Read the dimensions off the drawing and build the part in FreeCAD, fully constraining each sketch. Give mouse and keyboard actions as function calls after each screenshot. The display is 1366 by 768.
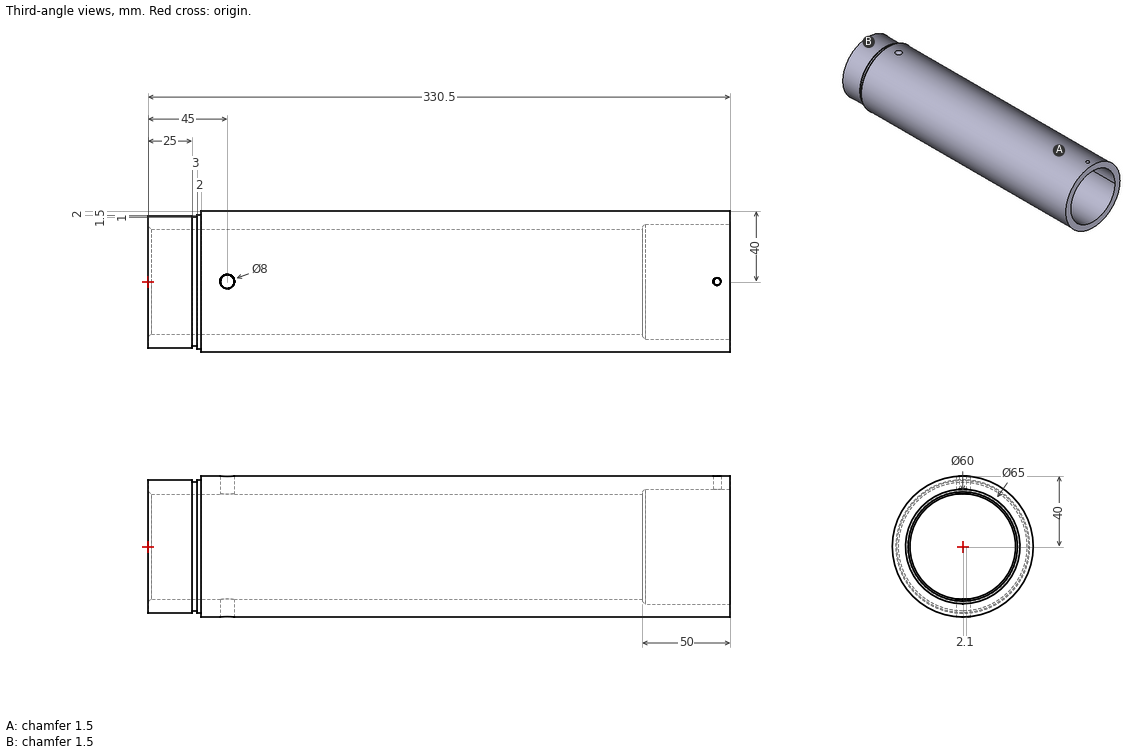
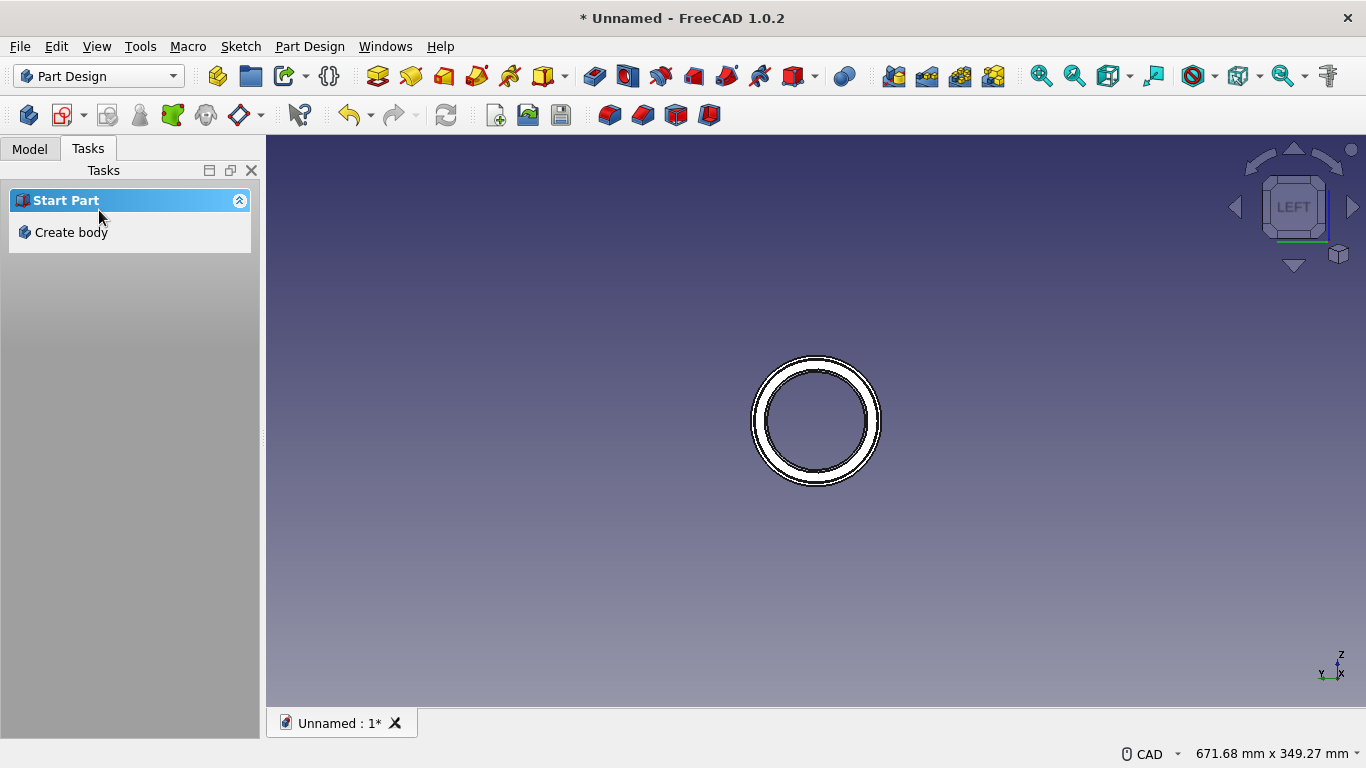
click(1042, 76)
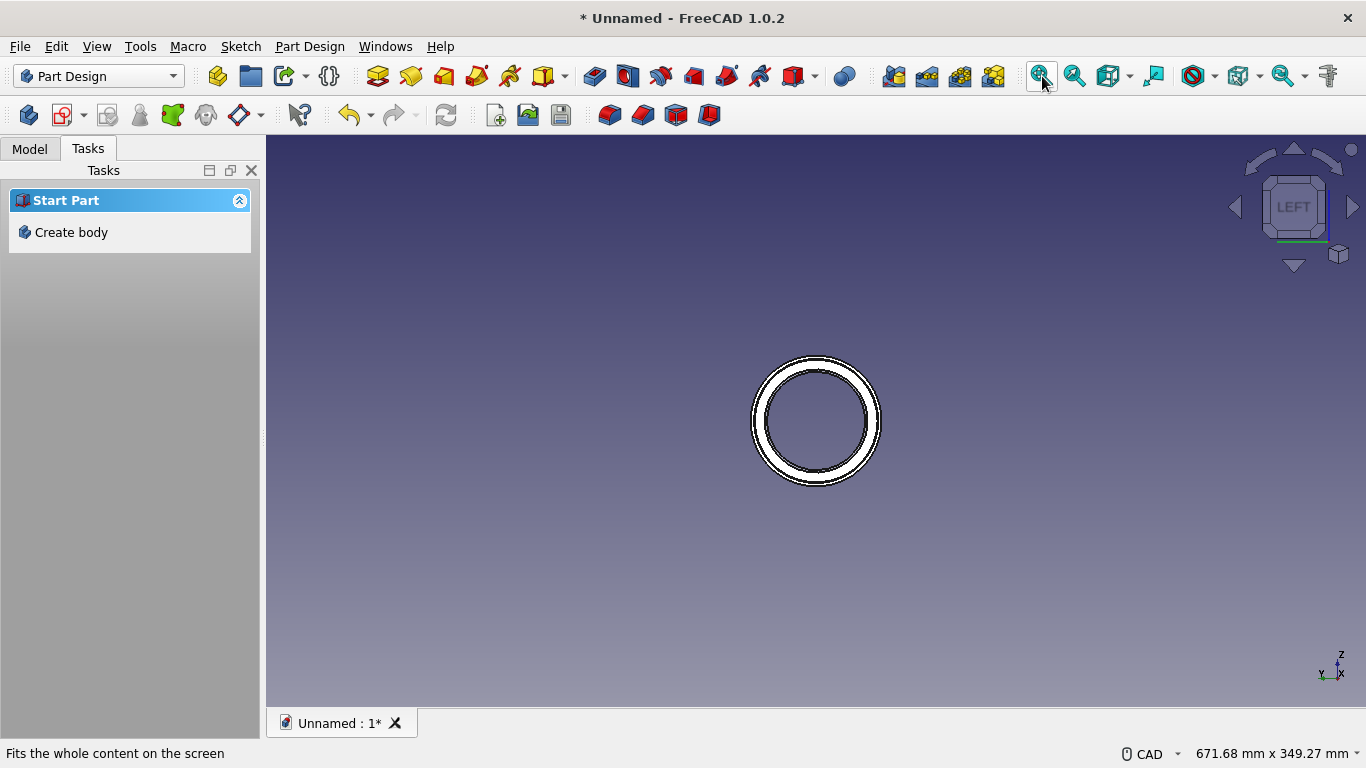
click(62, 116)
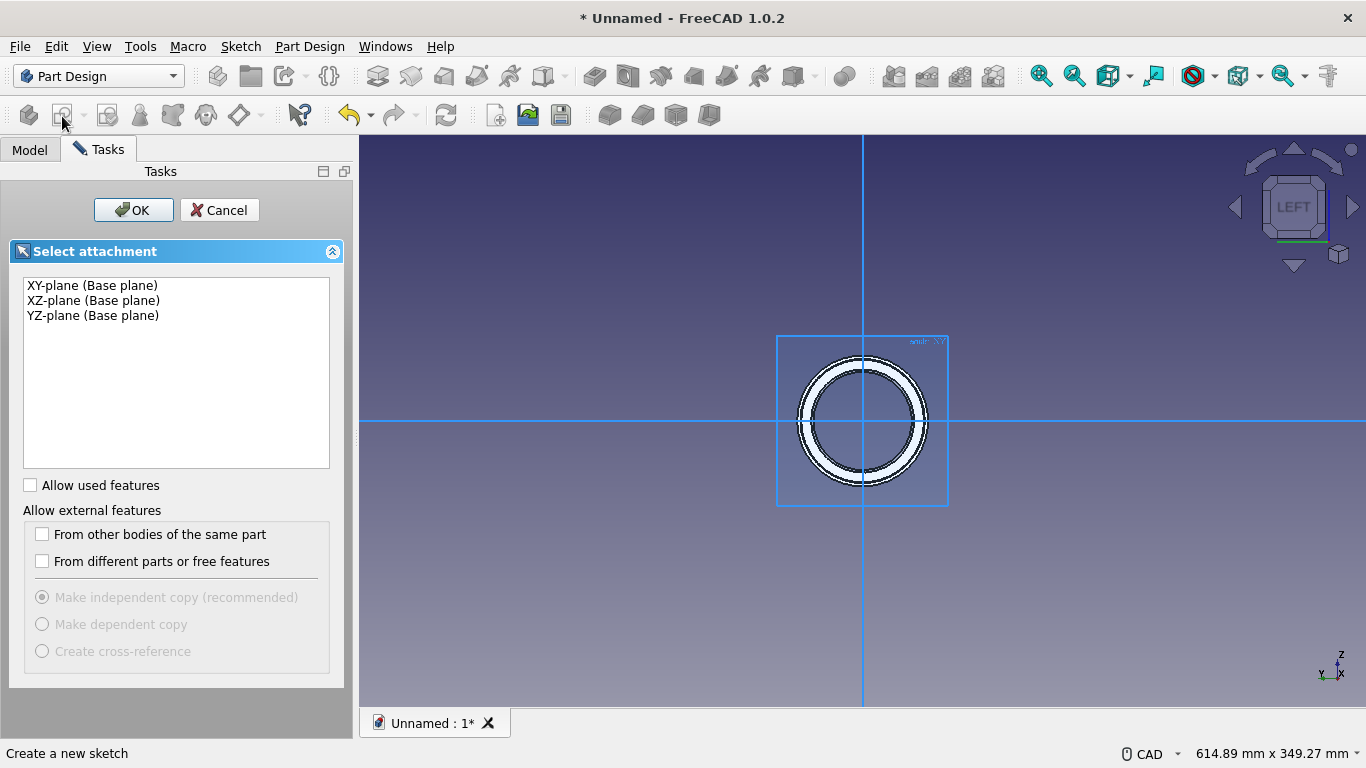
click(84, 286)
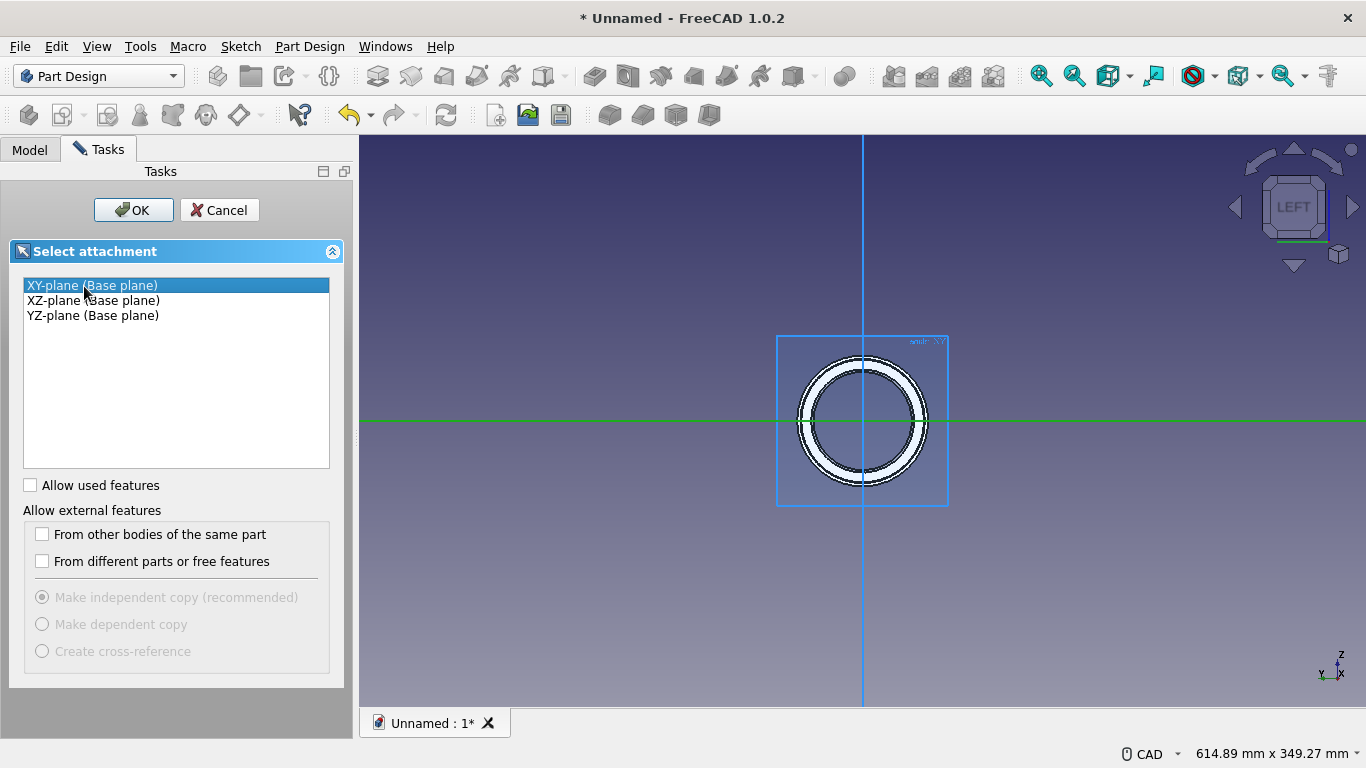
click(134, 210)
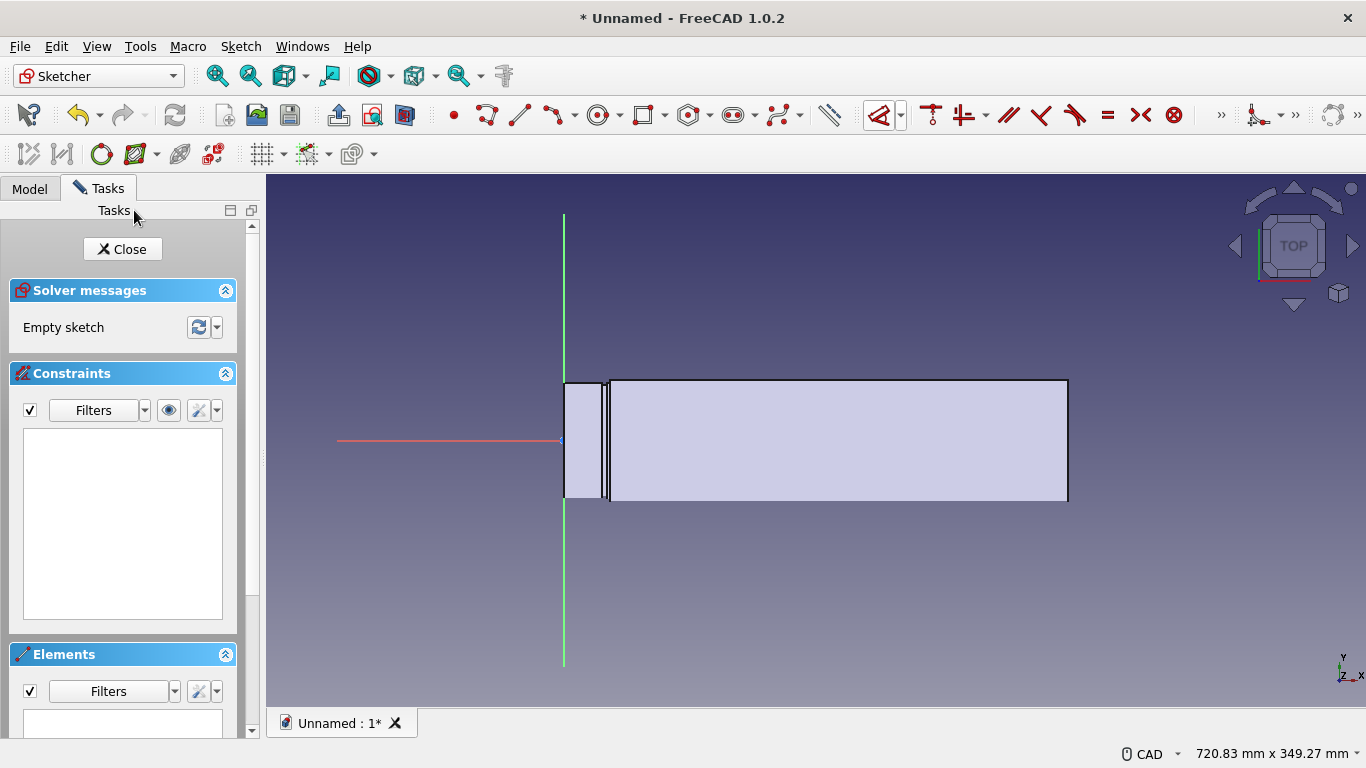
click(405, 116)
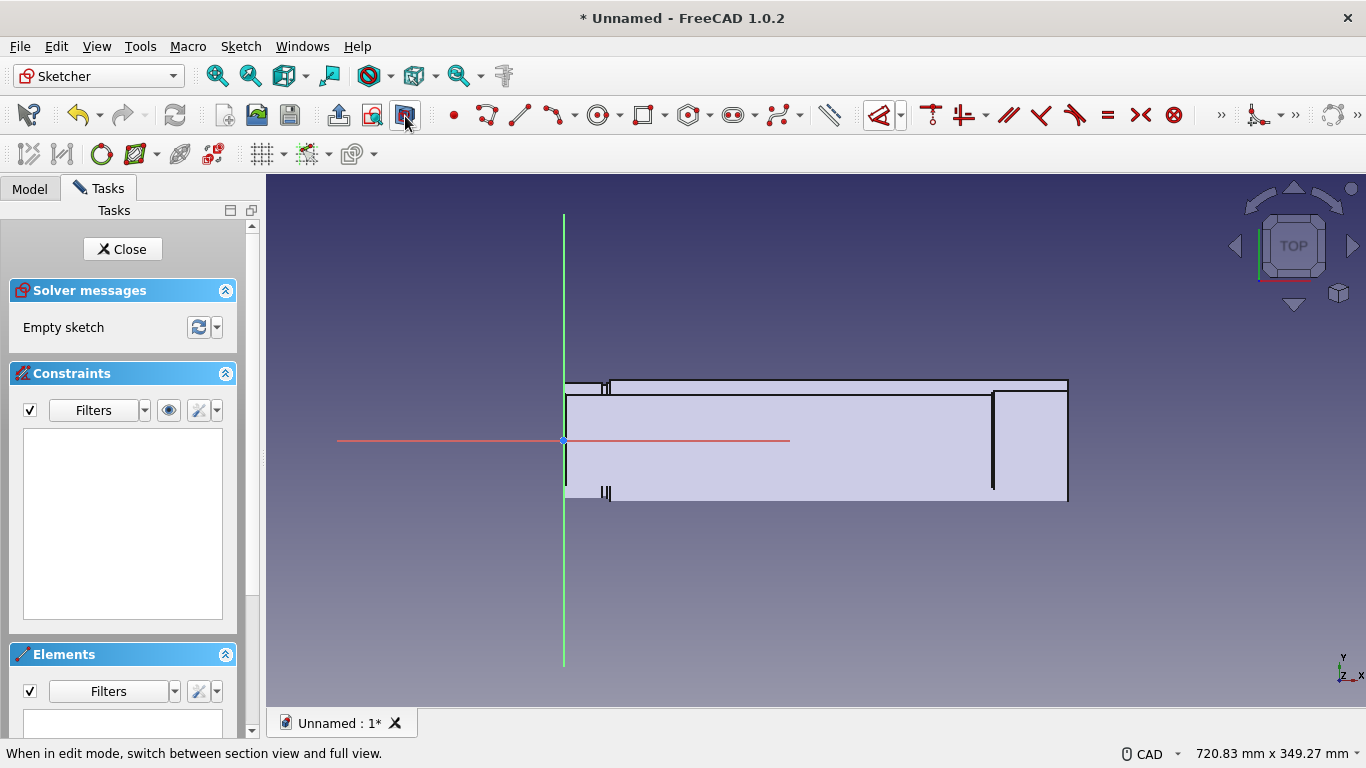
scroll(626, 441, up, 15)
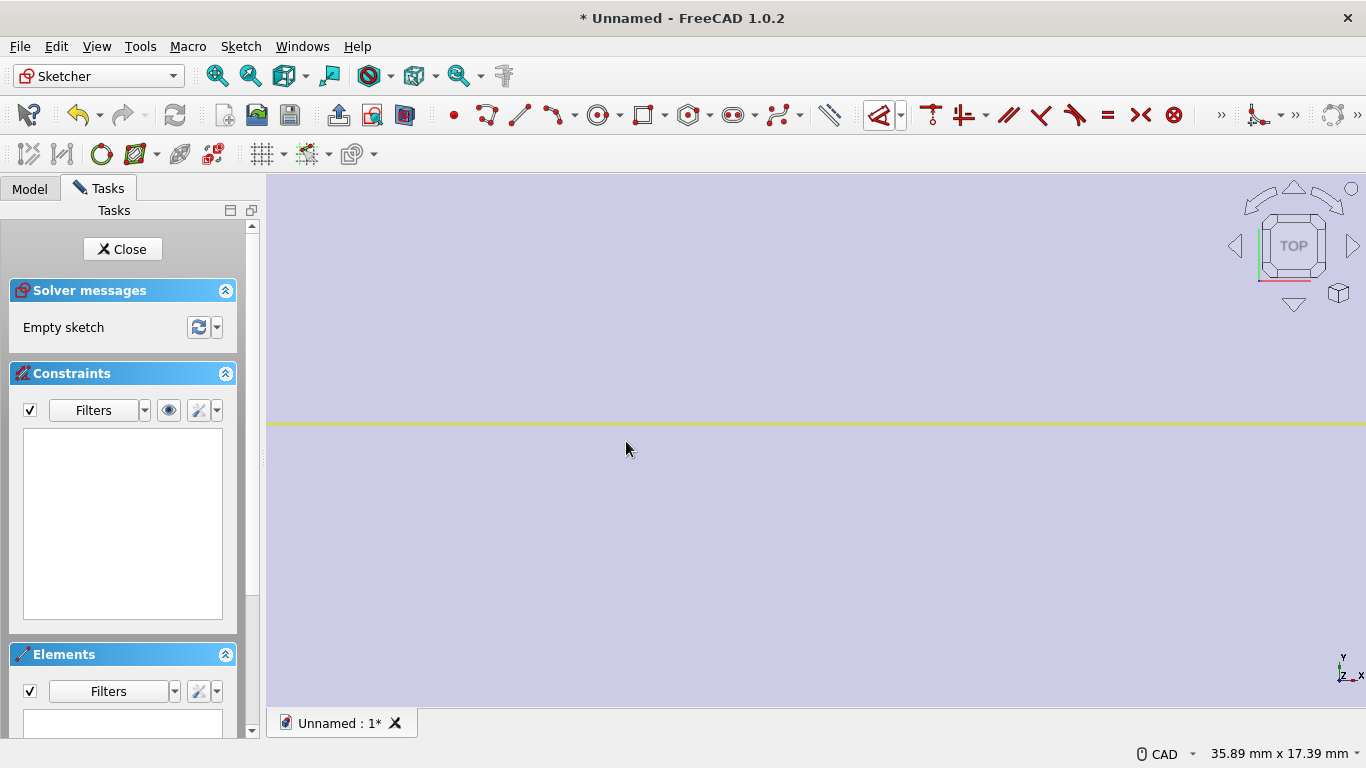
scroll(756, 390, up, 2)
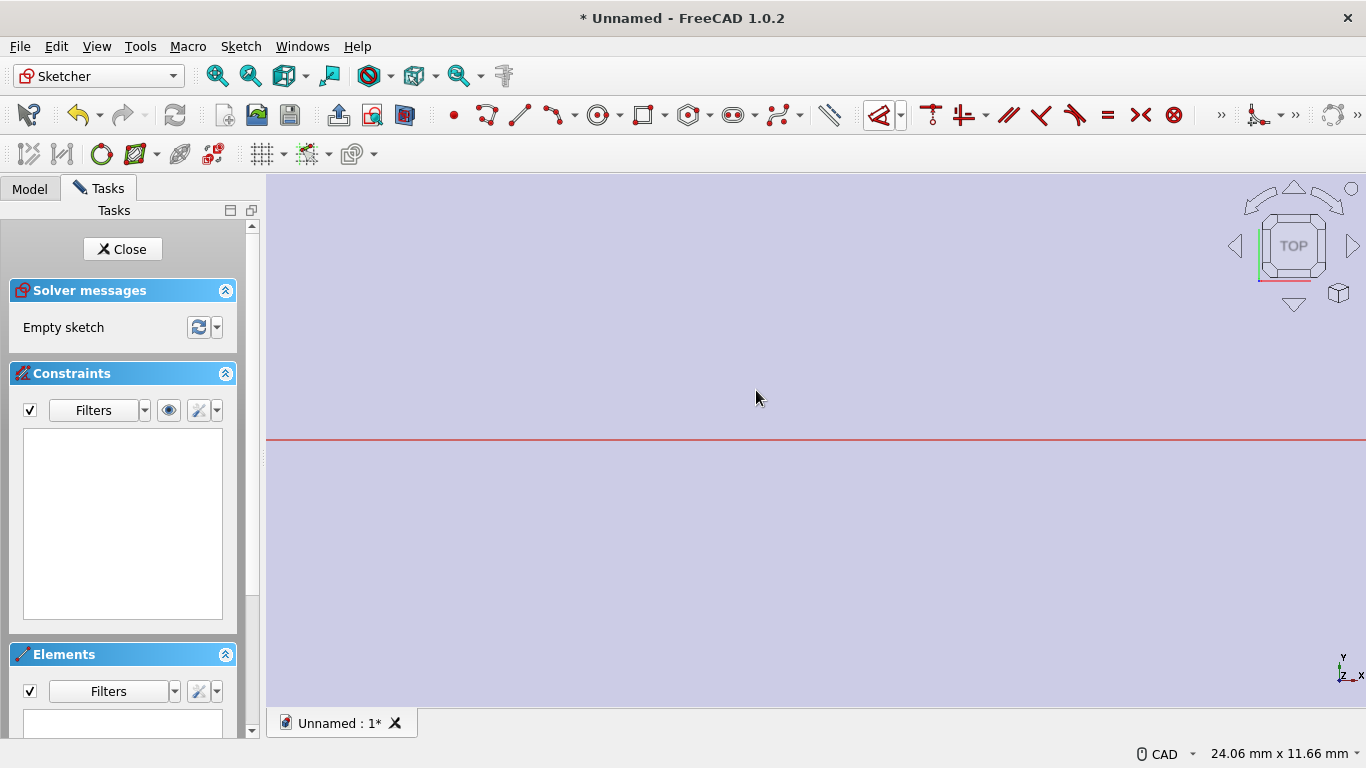
click(598, 116)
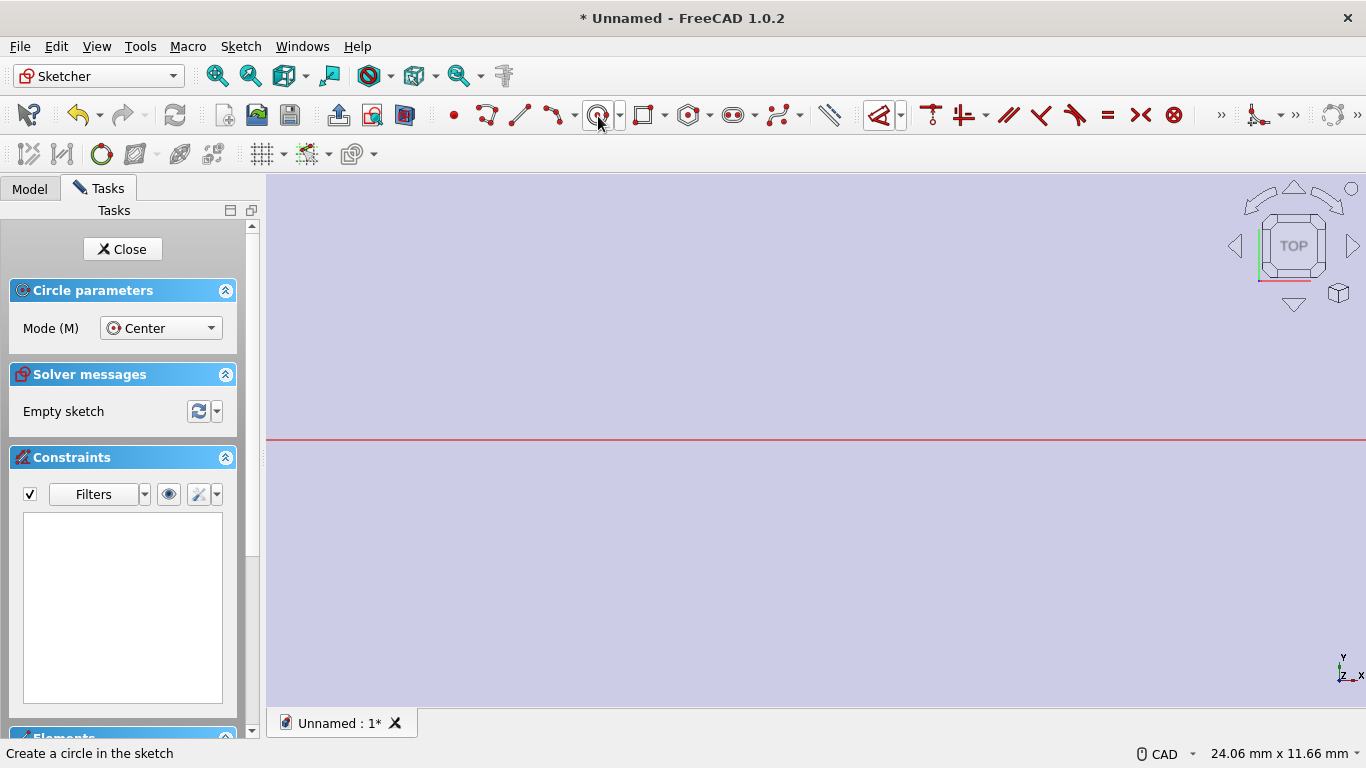
click(747, 440)
move(876, 311)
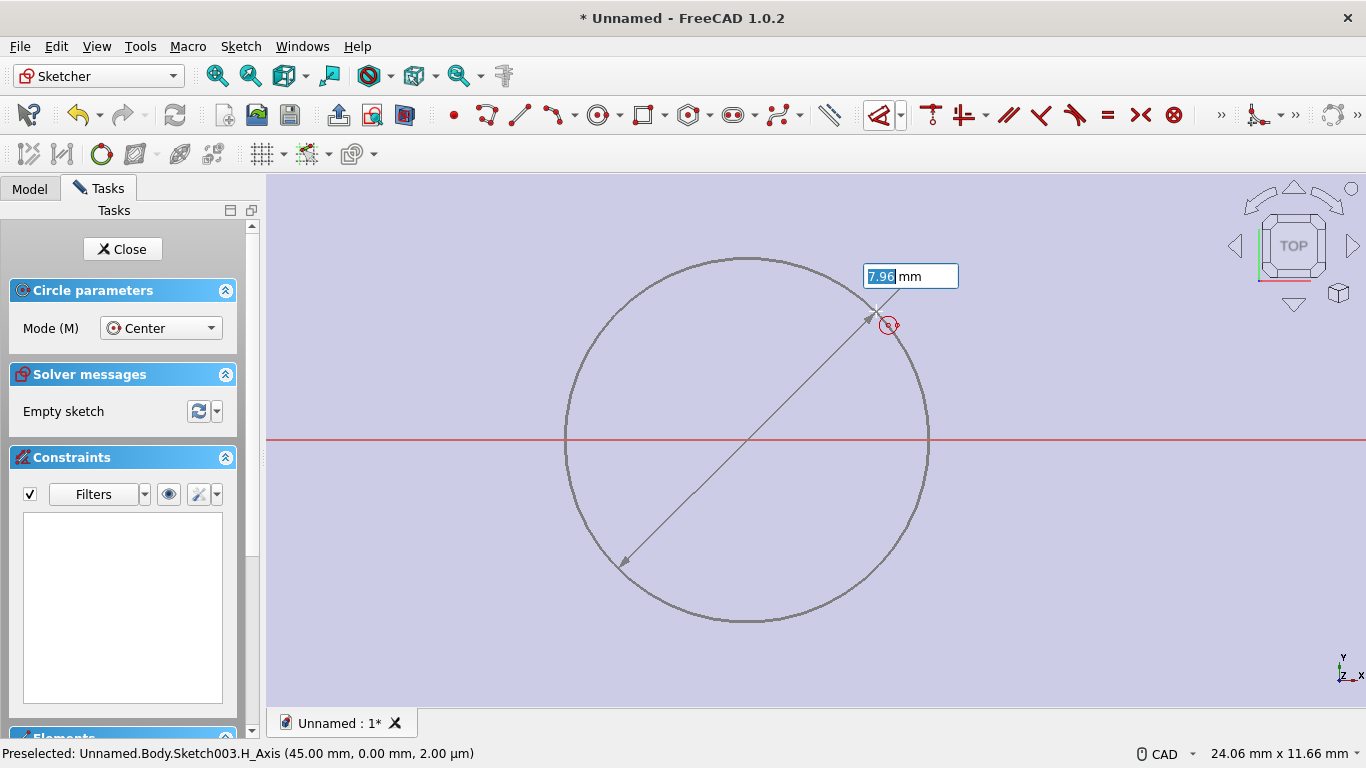
text(8)
key(Return)
key(Escape)